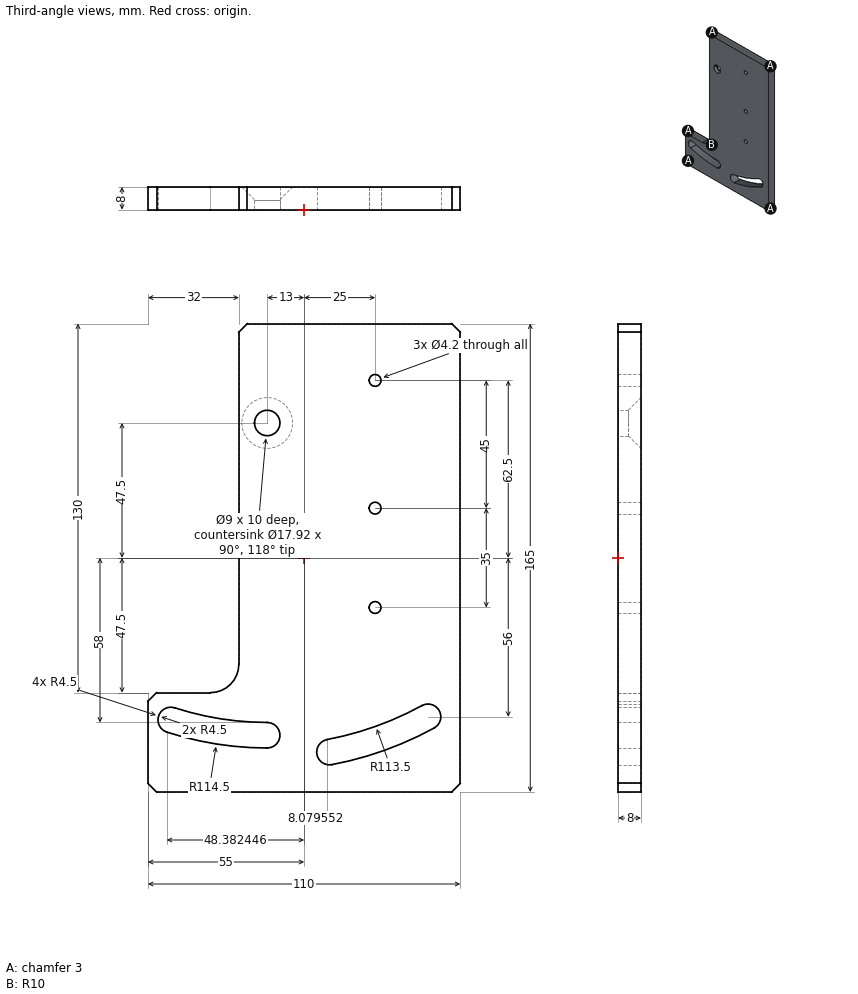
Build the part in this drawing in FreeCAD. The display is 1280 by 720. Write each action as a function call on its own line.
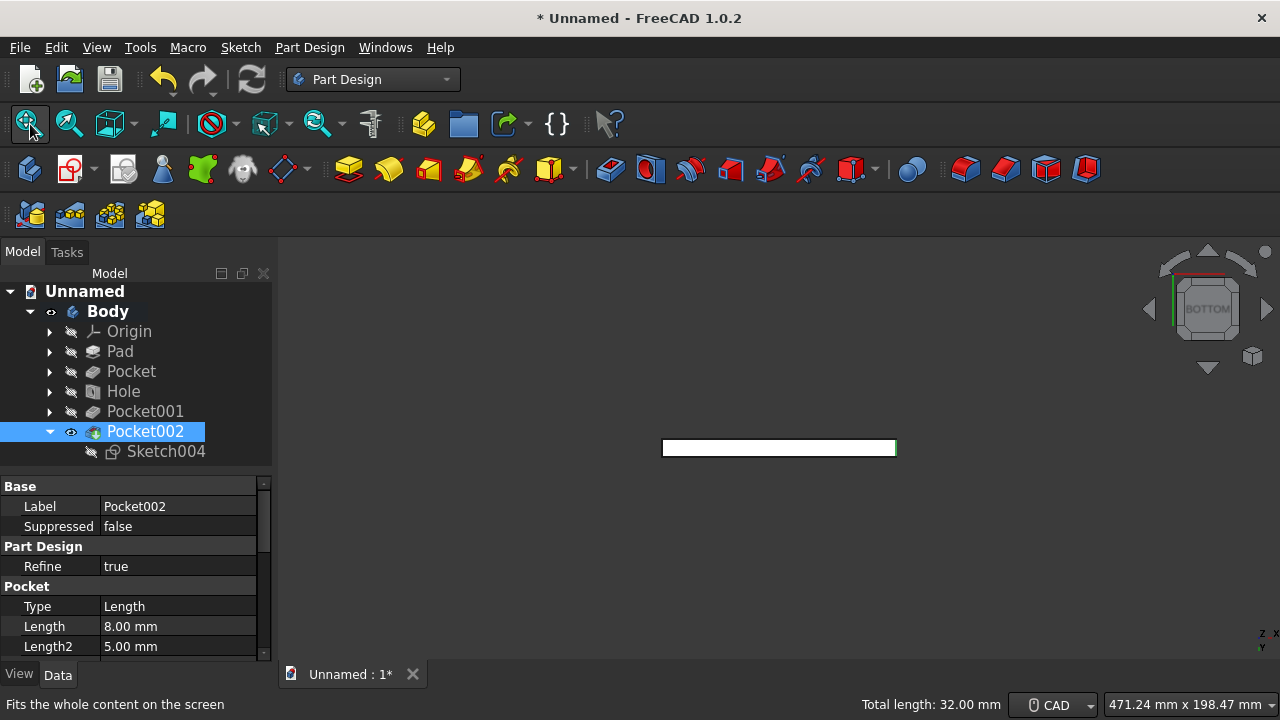
click(30, 124)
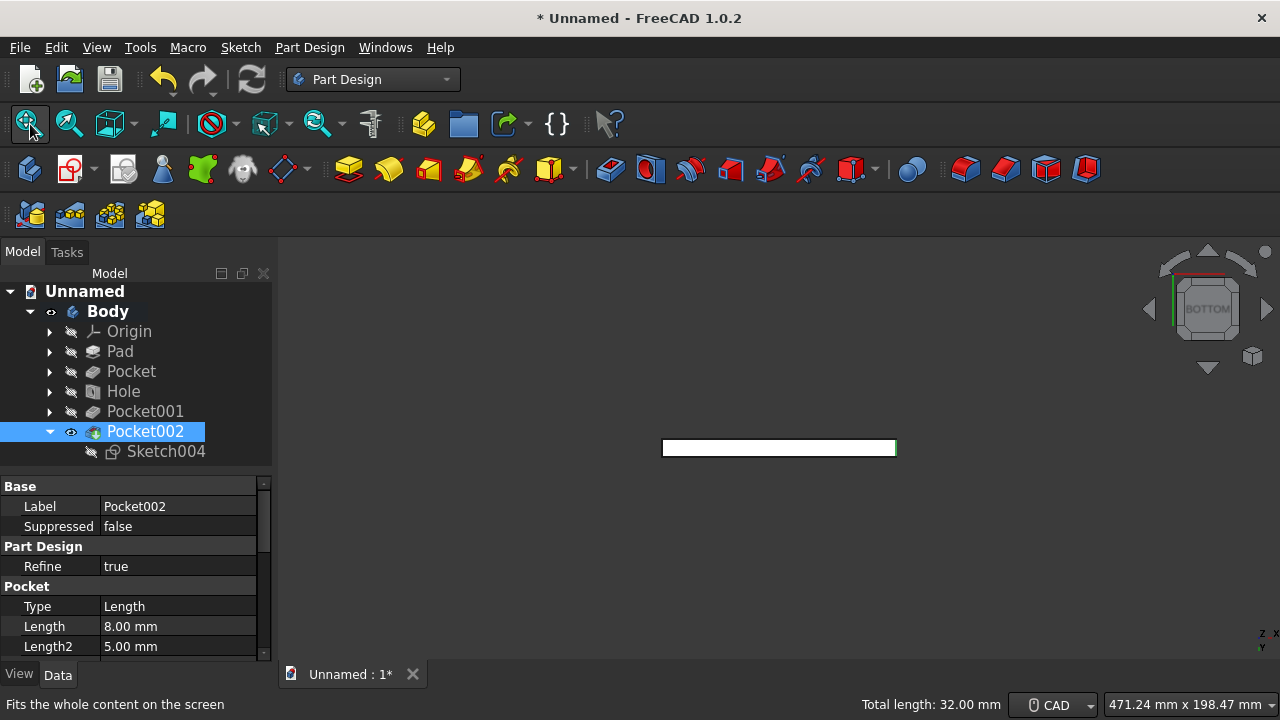
click(662, 447, ctrl)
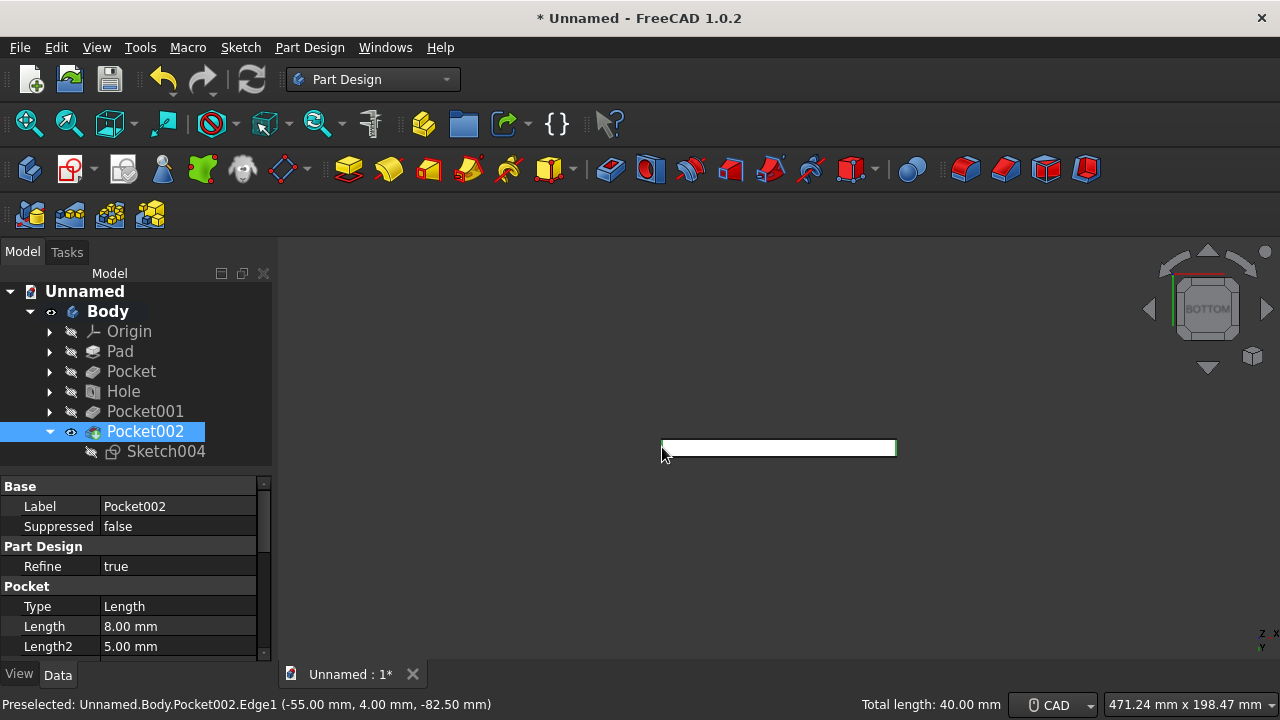
click(1006, 170)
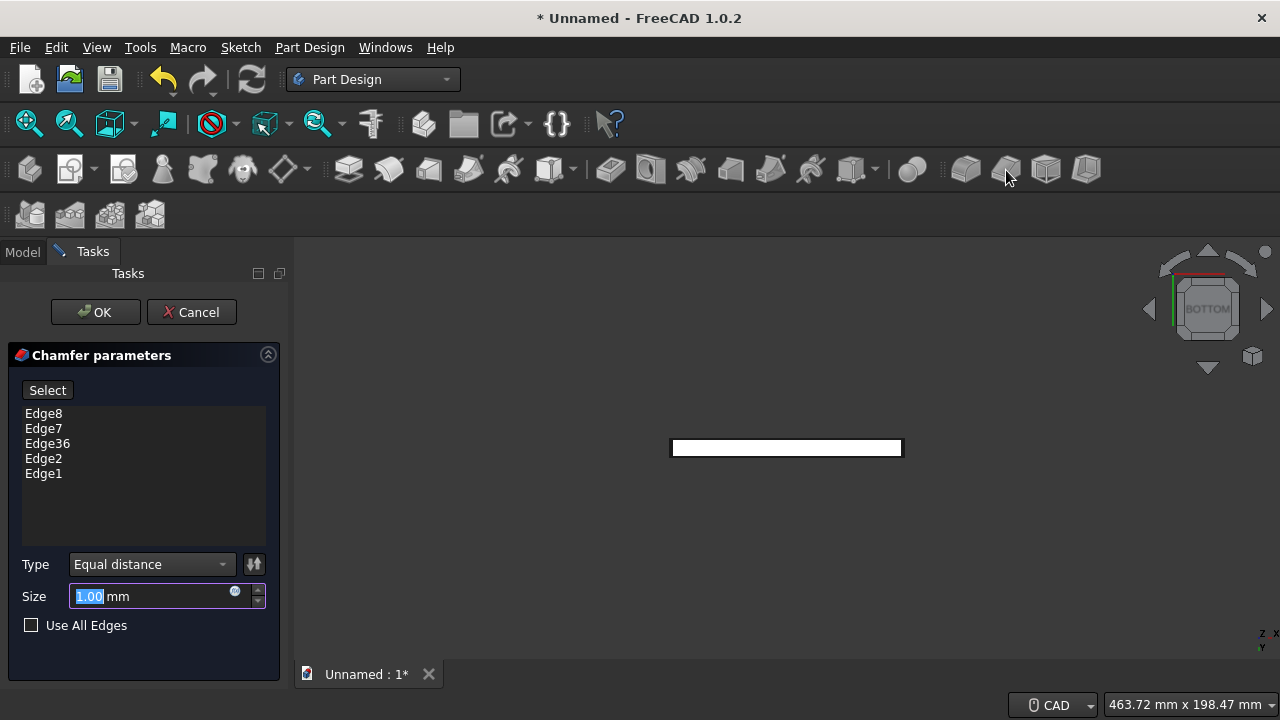
text(3)
key(Tab)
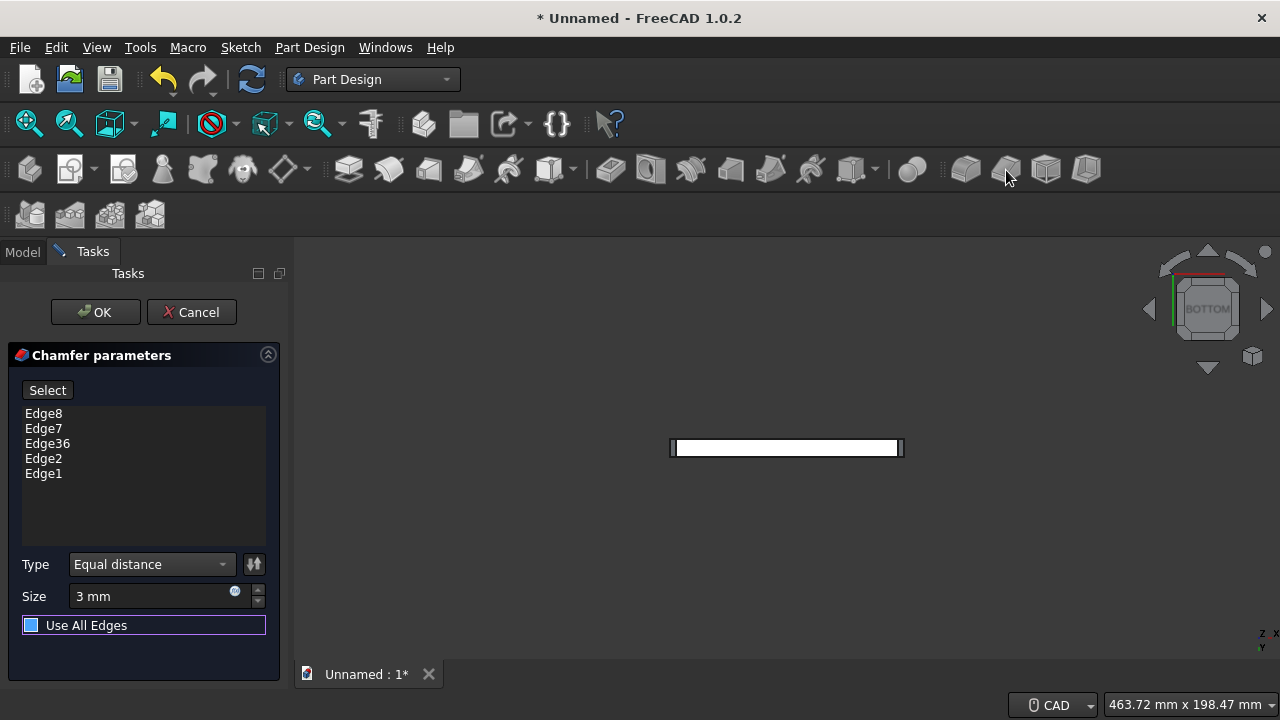
click(96, 312)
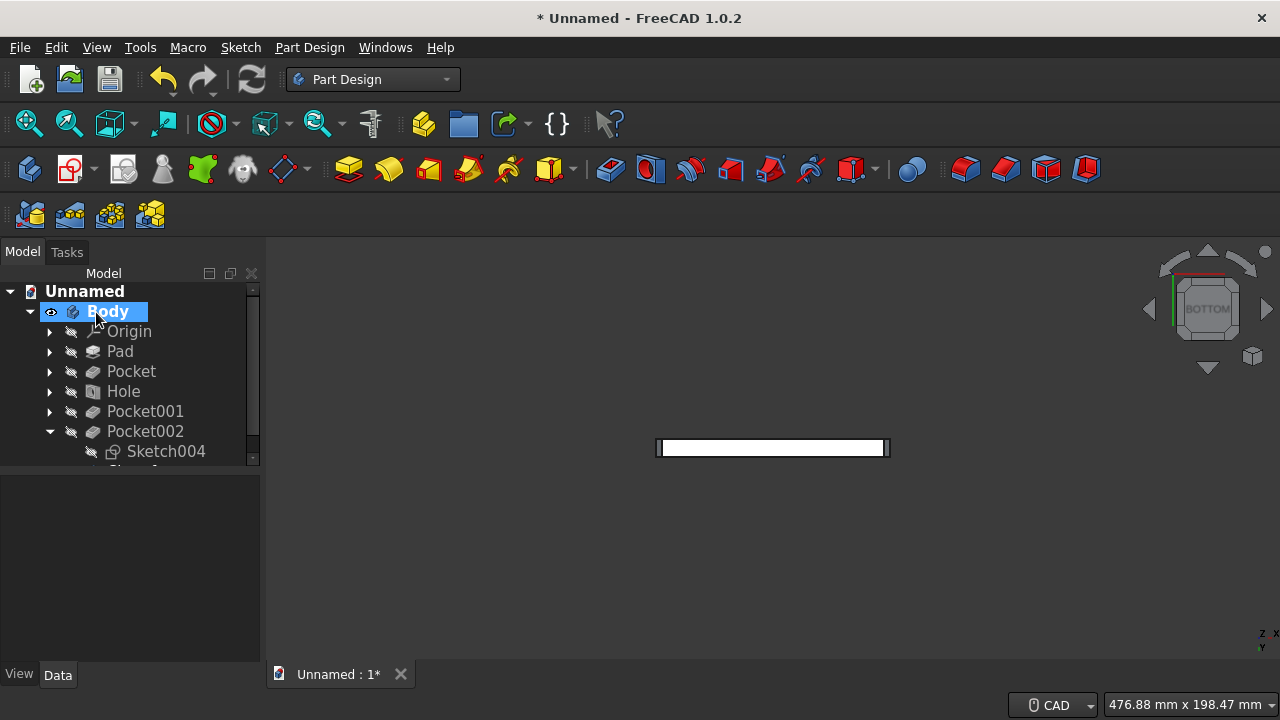
click(30, 124)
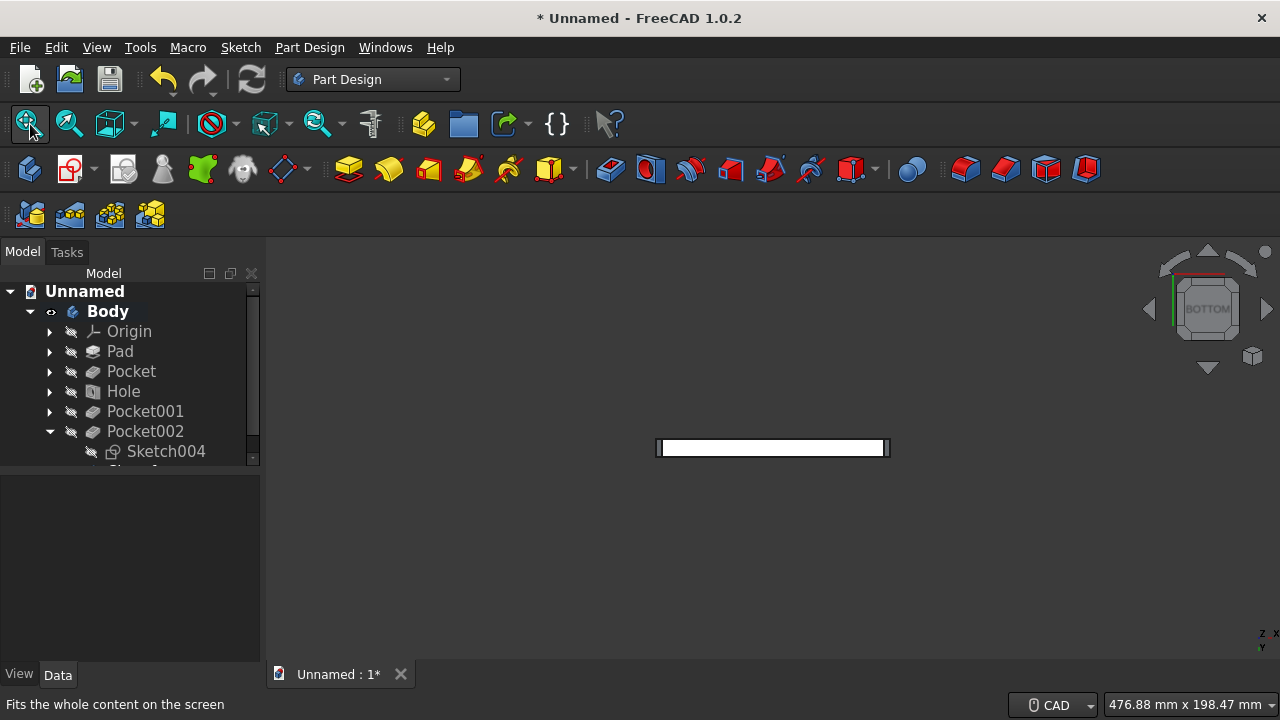
key(4)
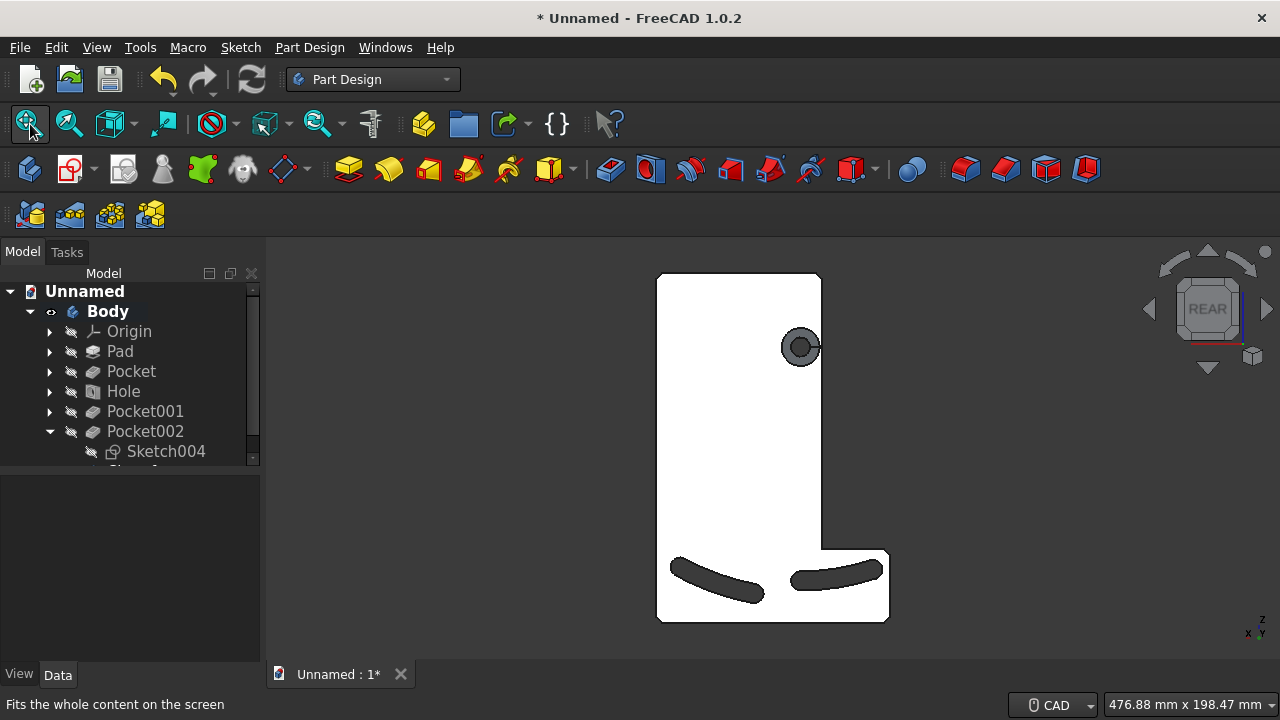
click(740, 447)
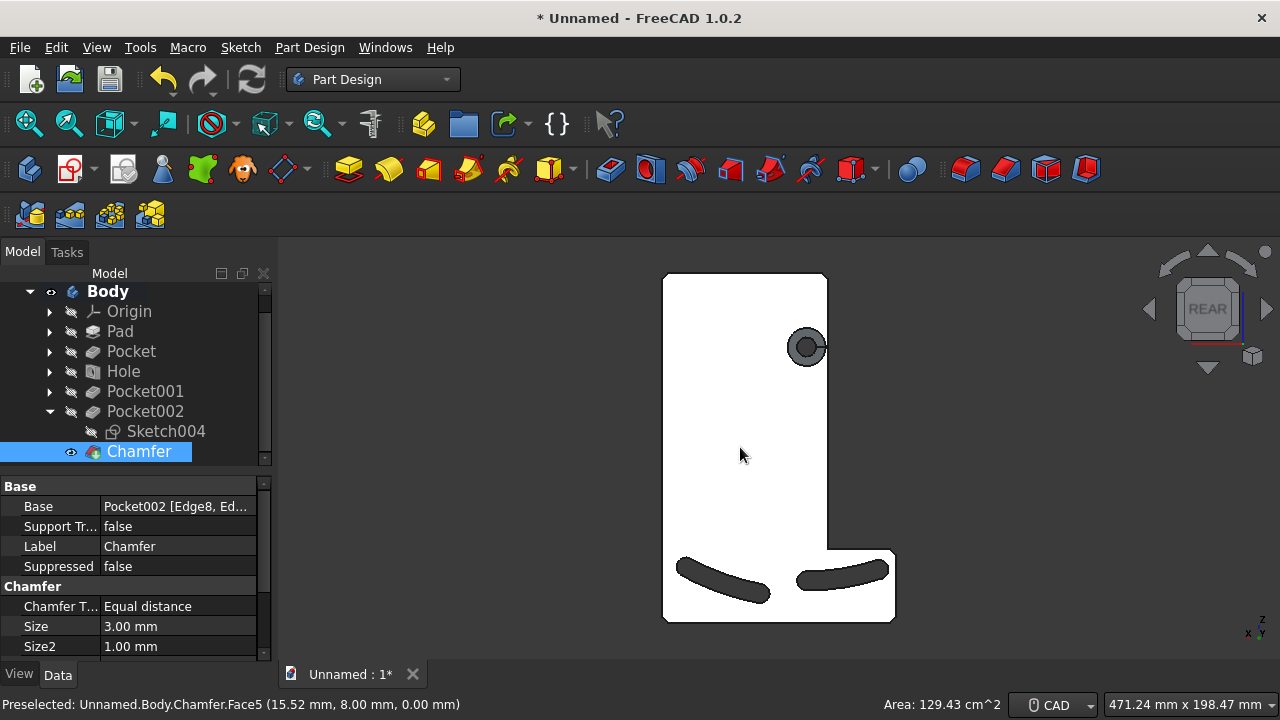
click(70, 170)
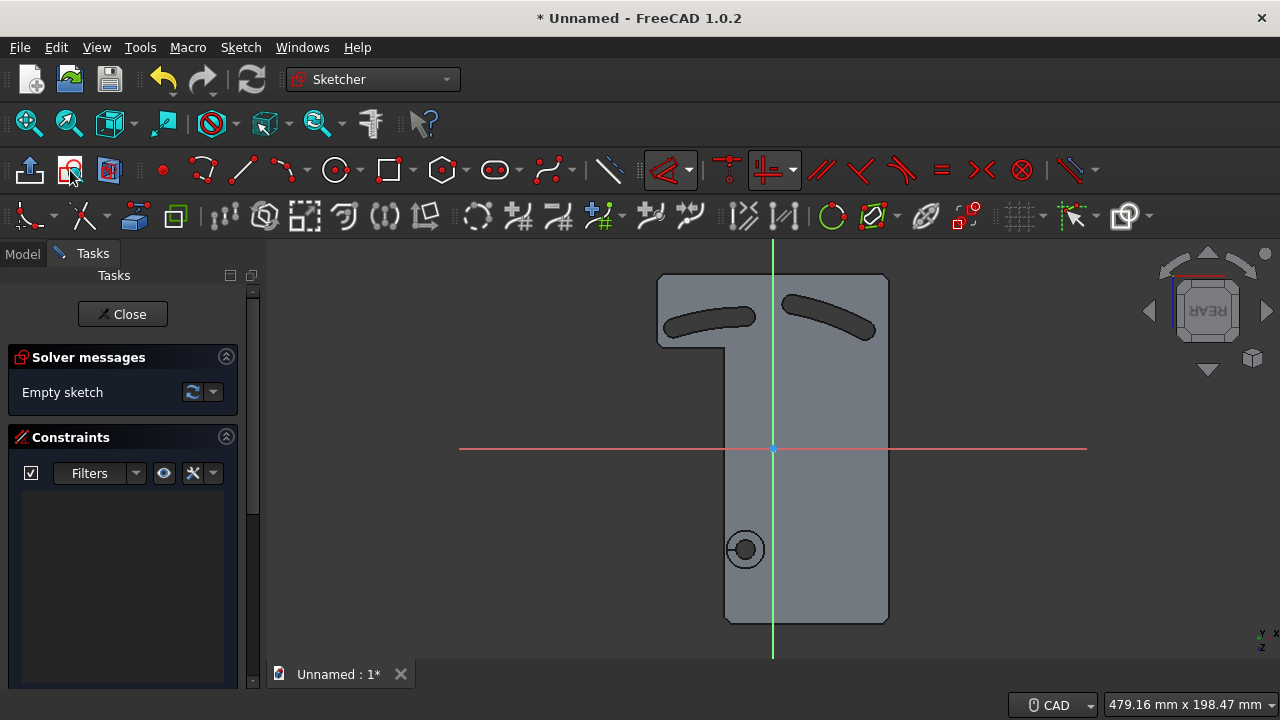
scroll(999, 593, up, 2)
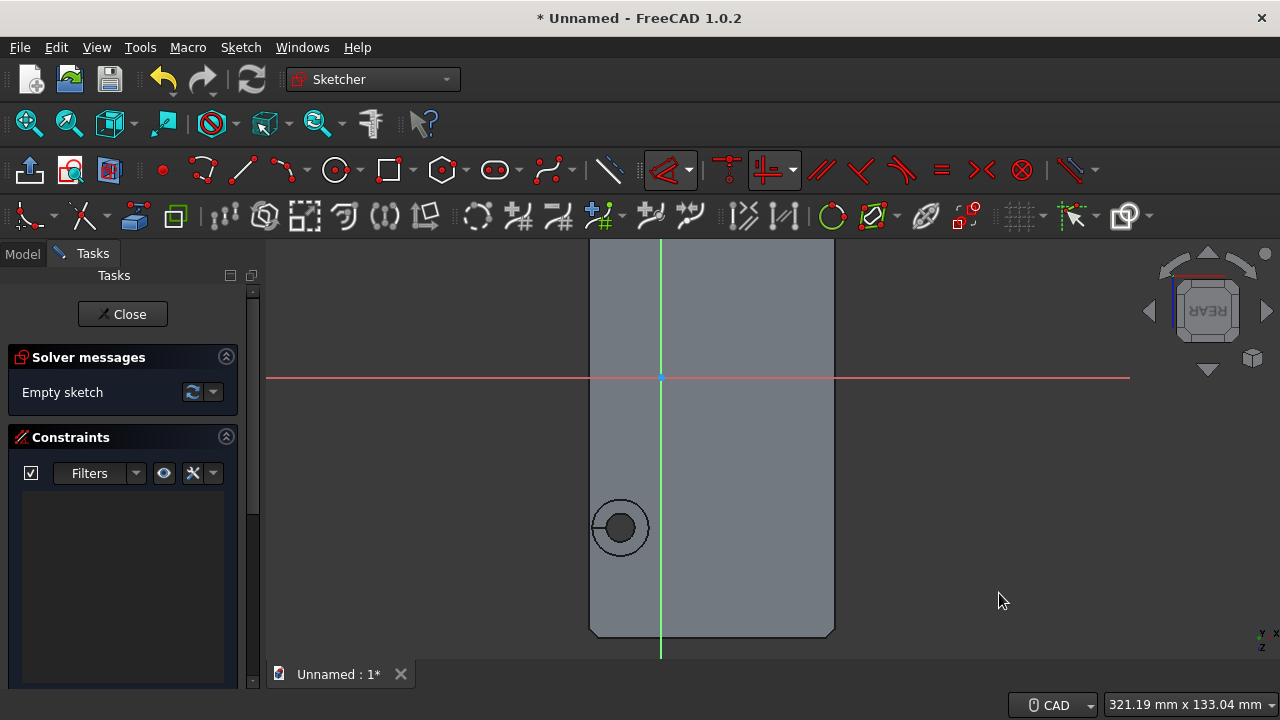
click(336, 170)